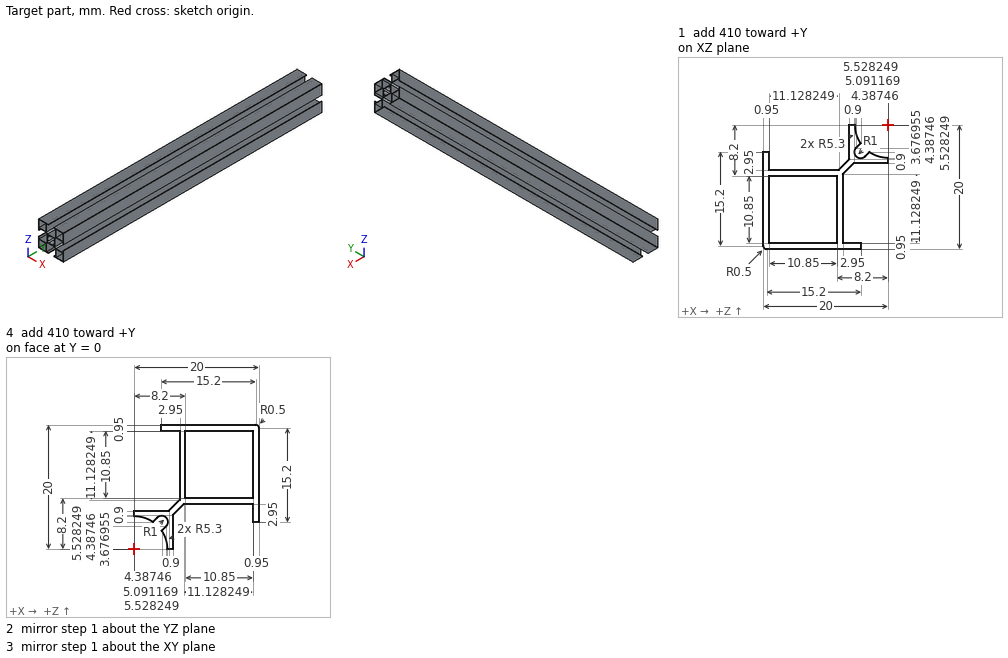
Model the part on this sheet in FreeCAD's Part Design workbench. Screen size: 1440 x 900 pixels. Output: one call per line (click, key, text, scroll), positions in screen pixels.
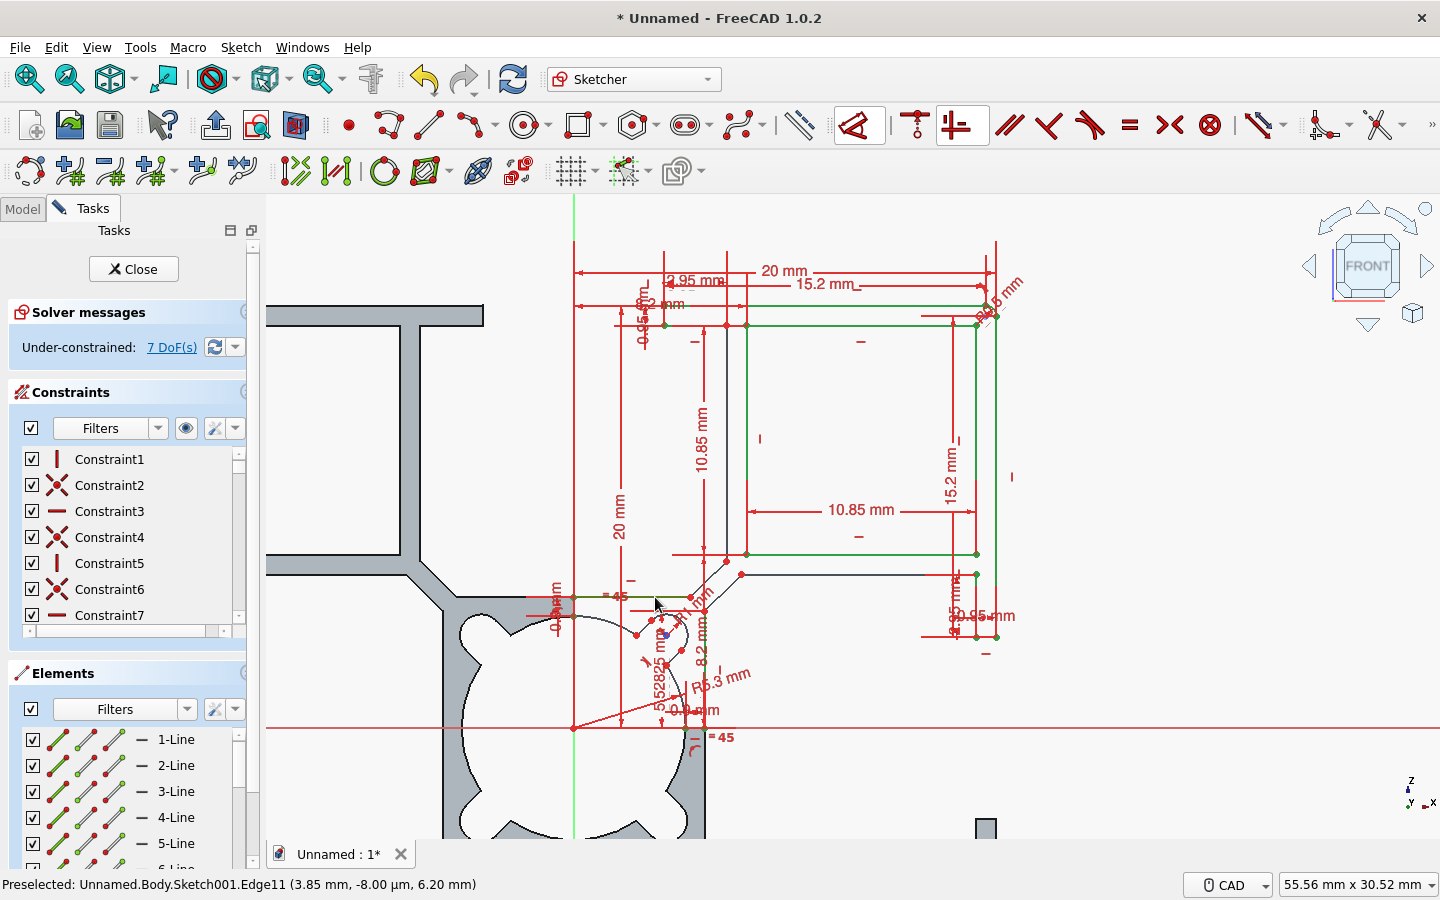
key(l)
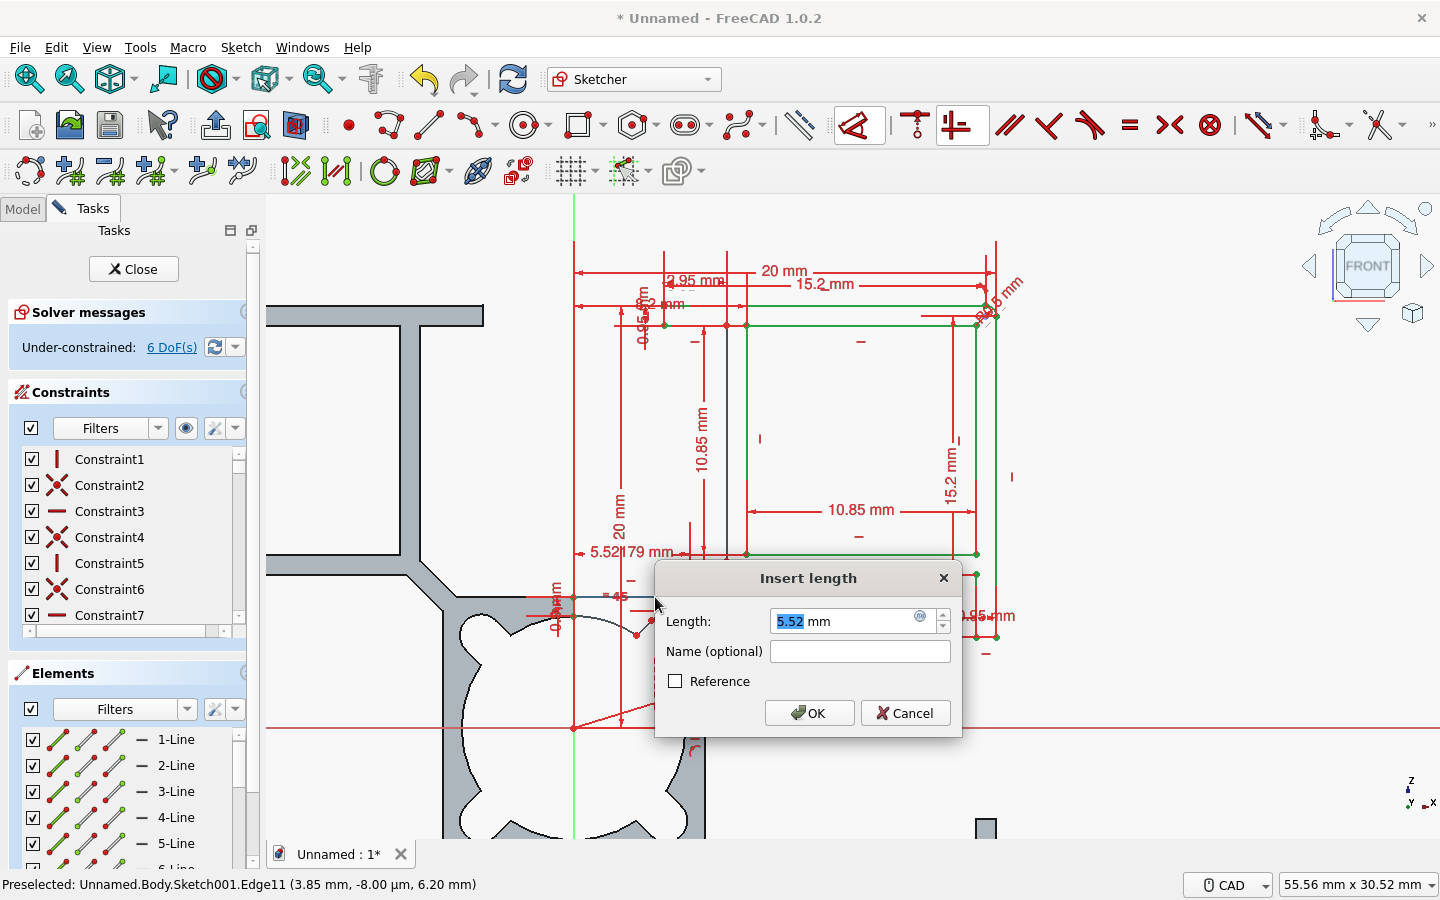
text(5.528249)
key(Return)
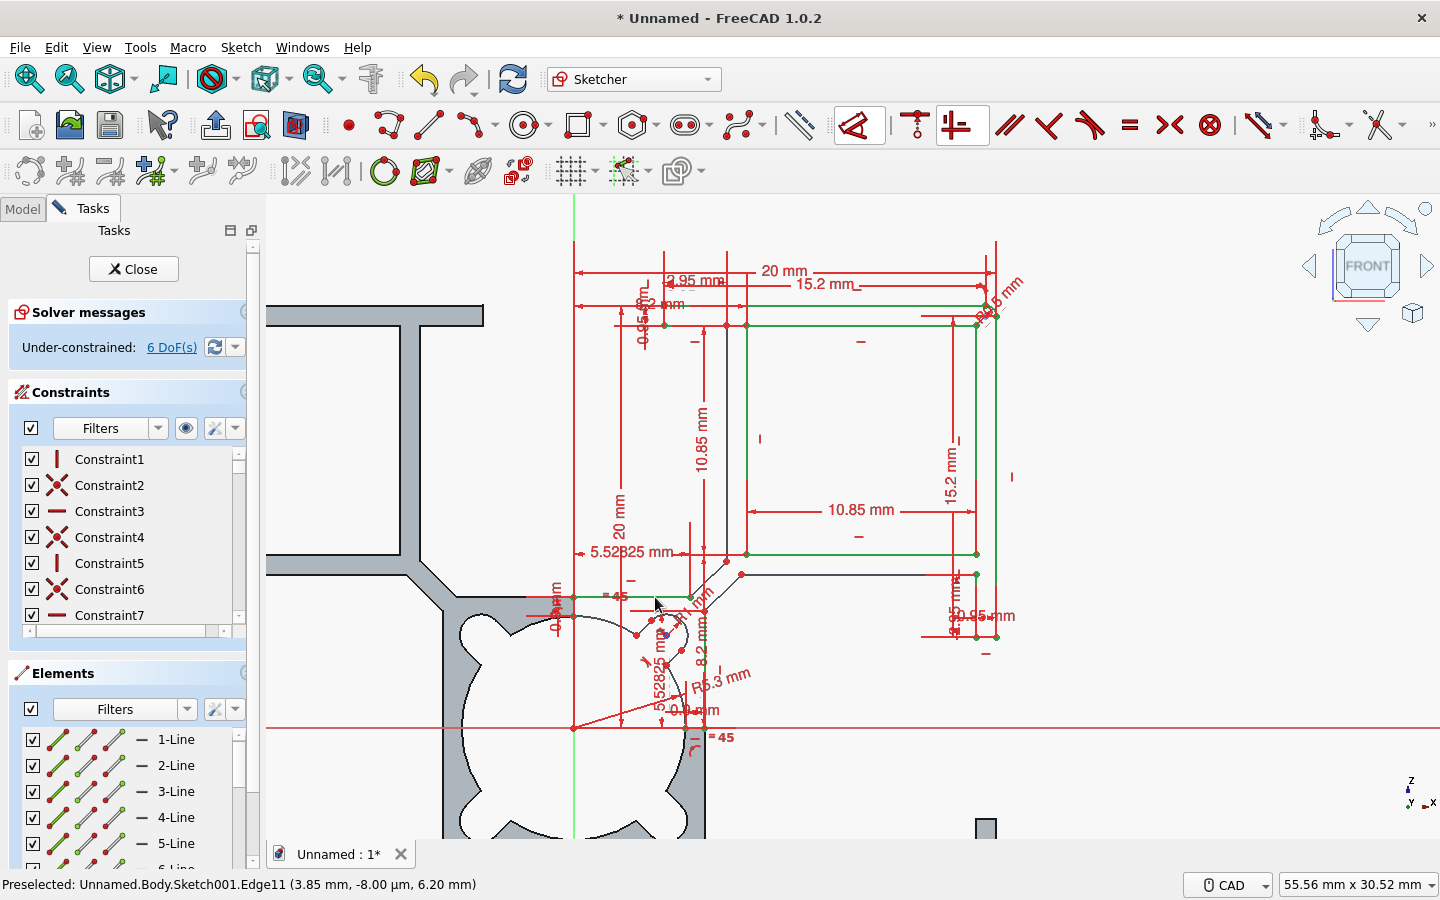
click(666, 665)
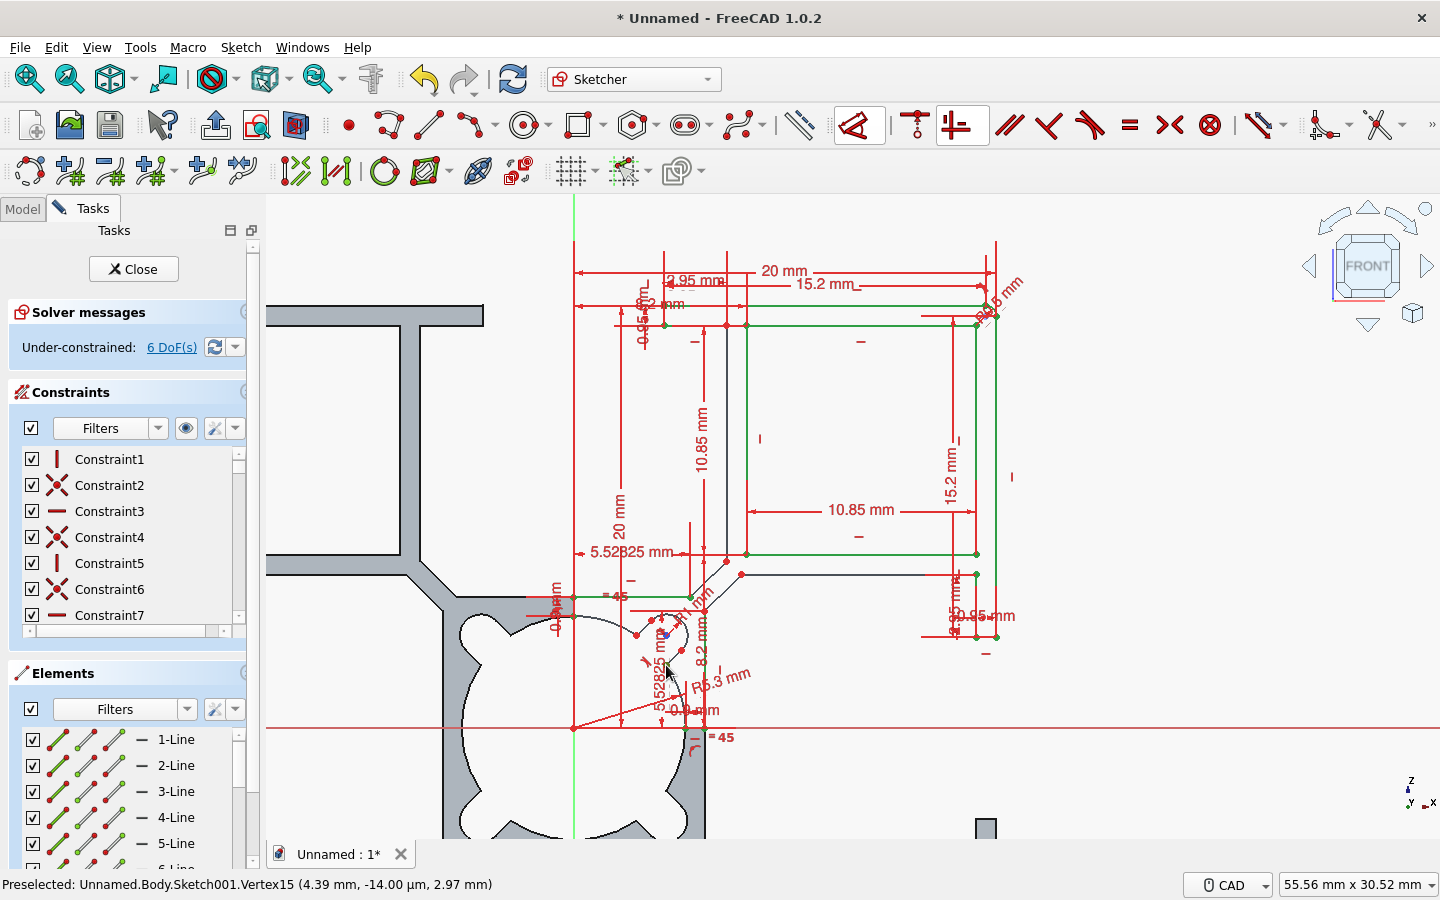
key(l)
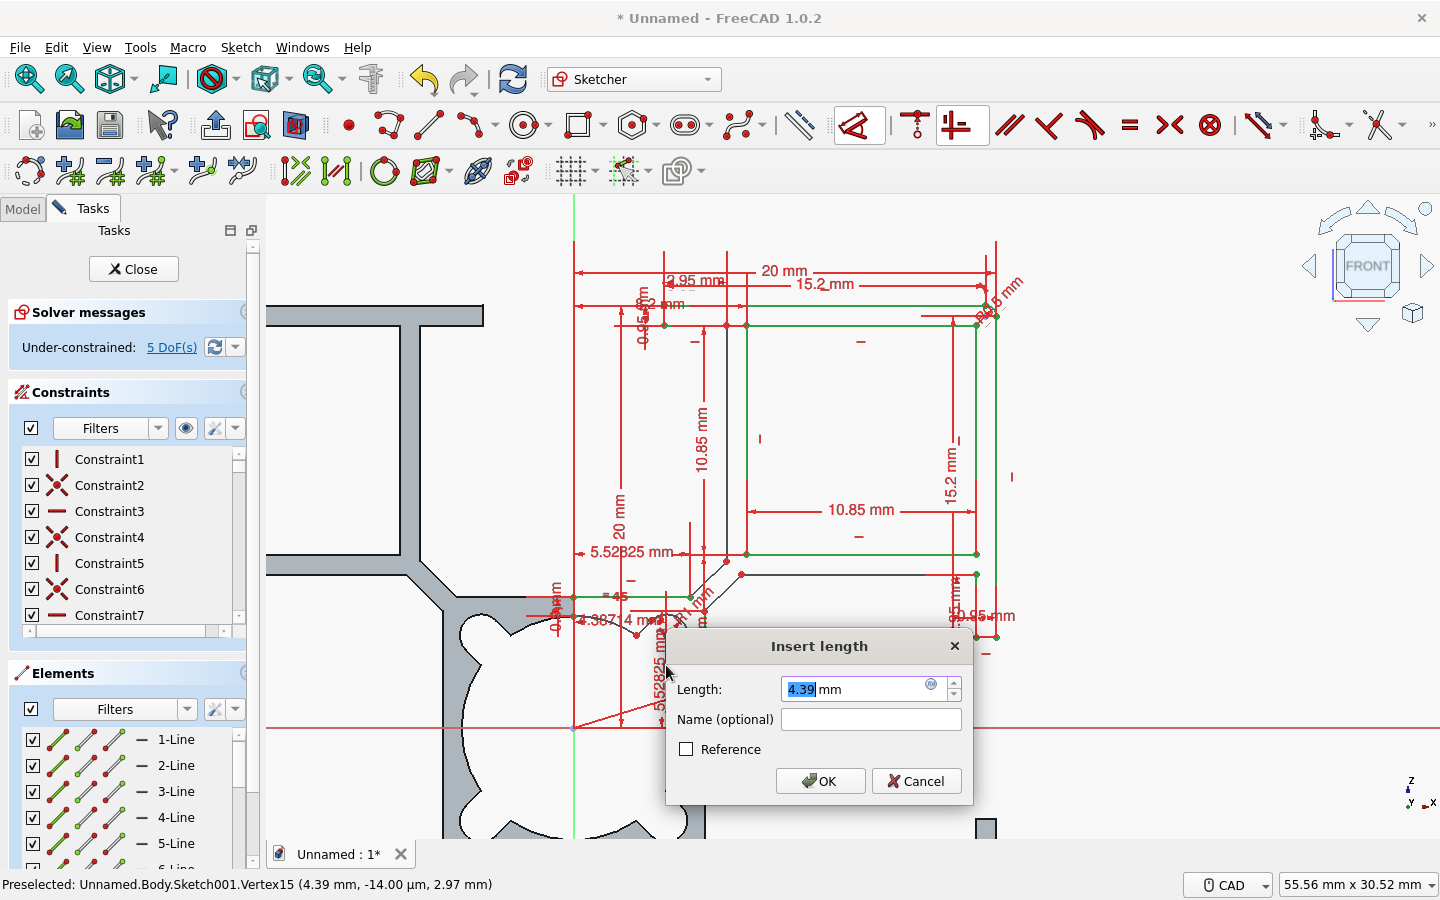
text(4.38746)
key(Return)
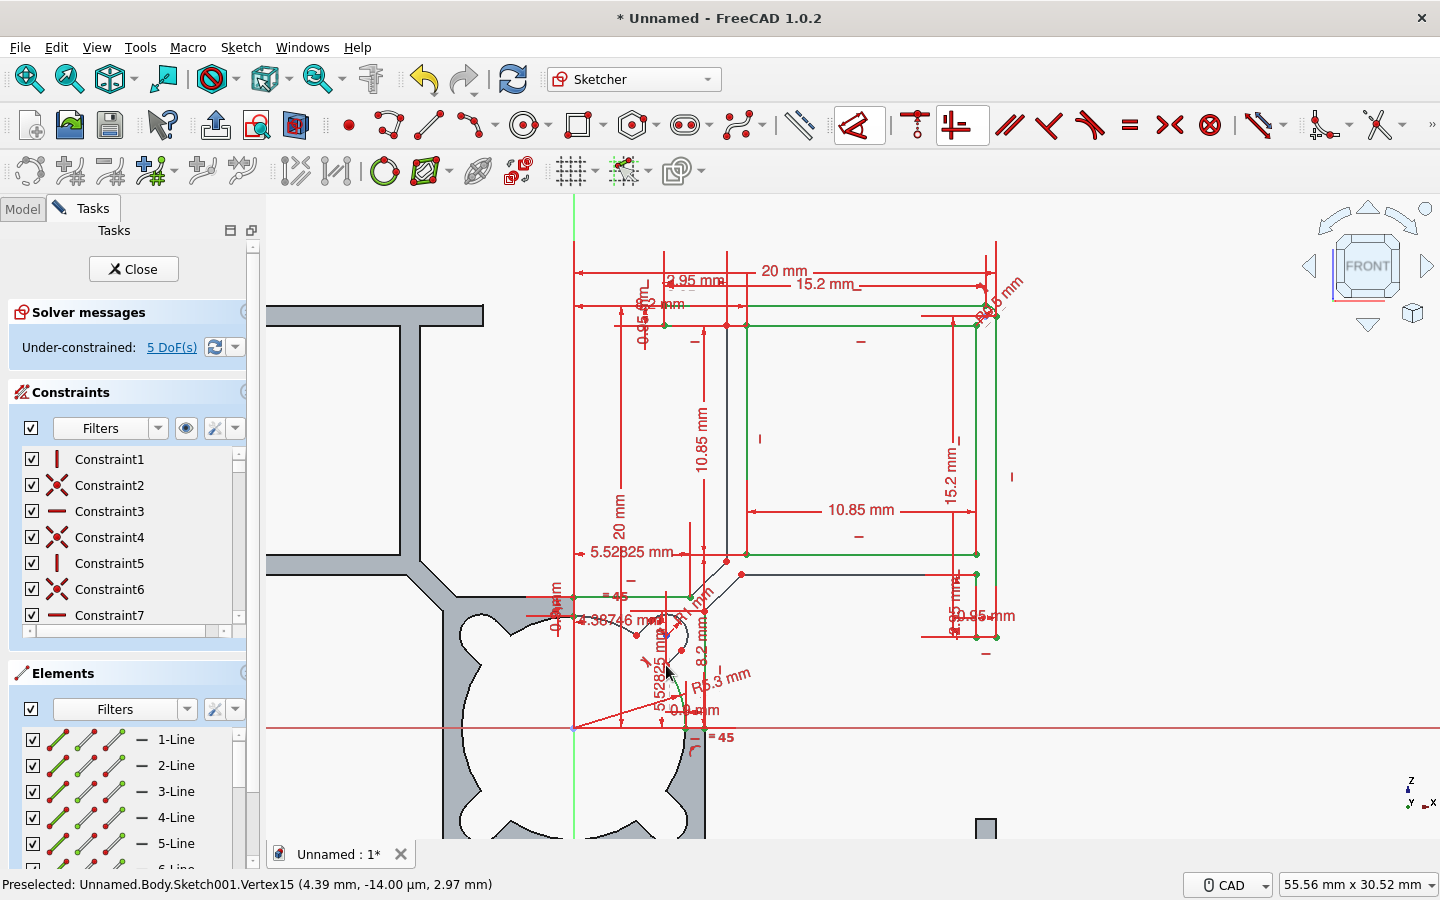
click(637, 636)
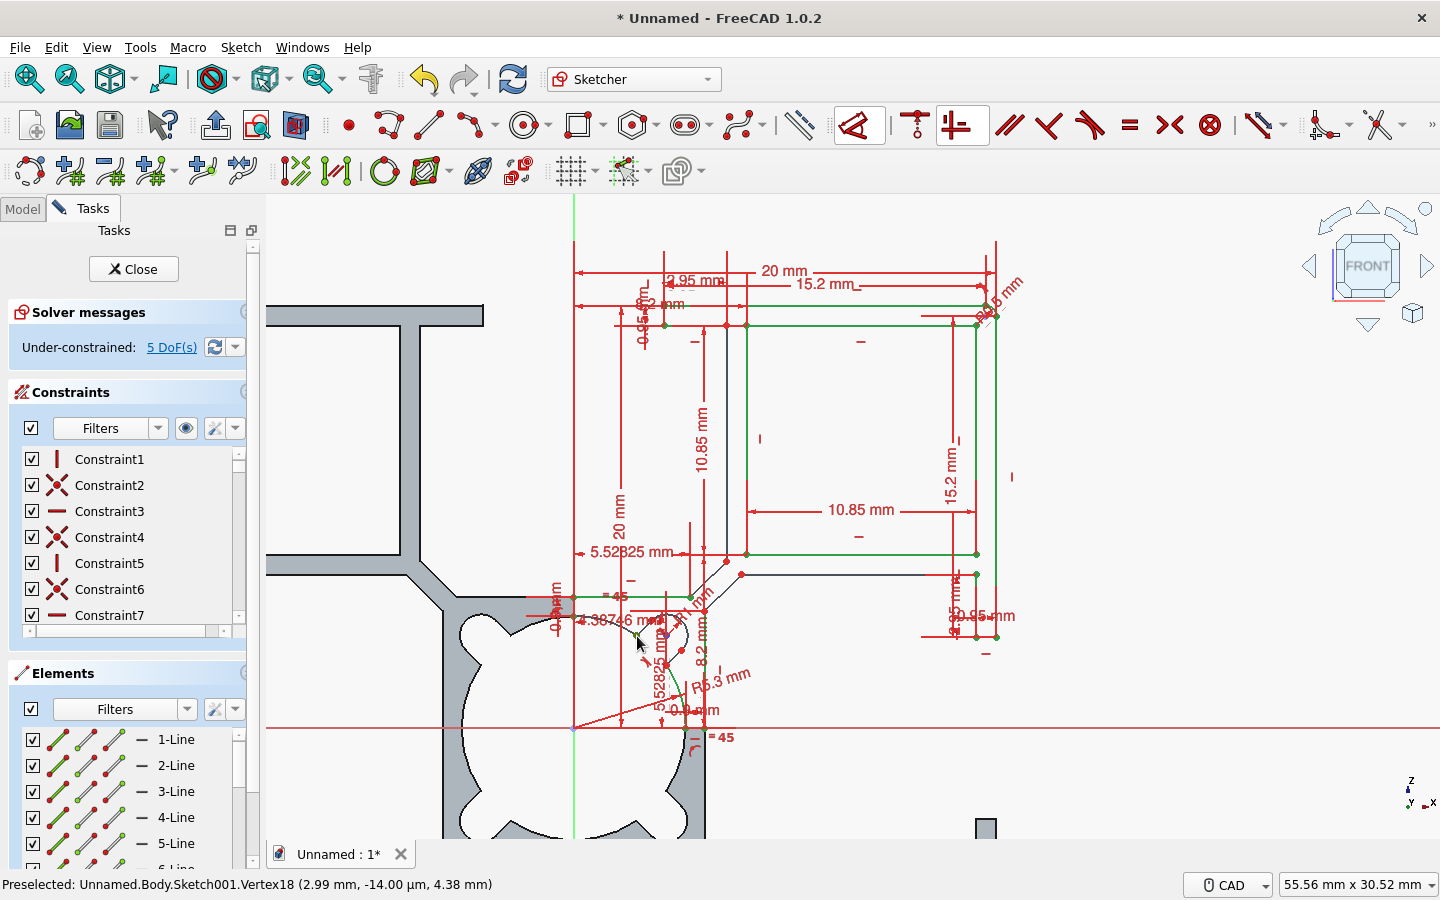
key(i)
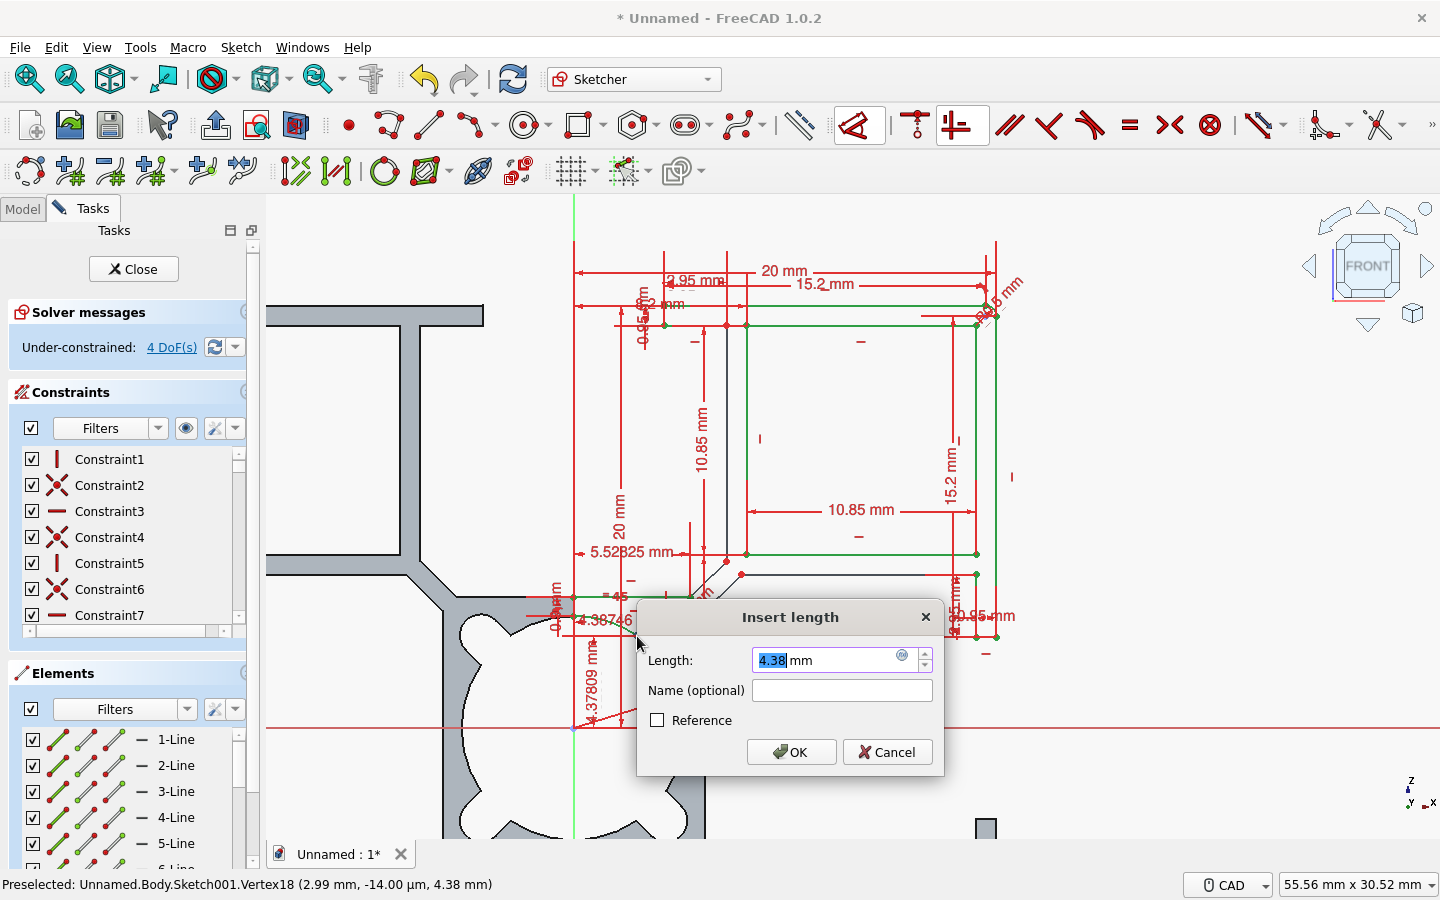
text(4.38746)
key(Return)